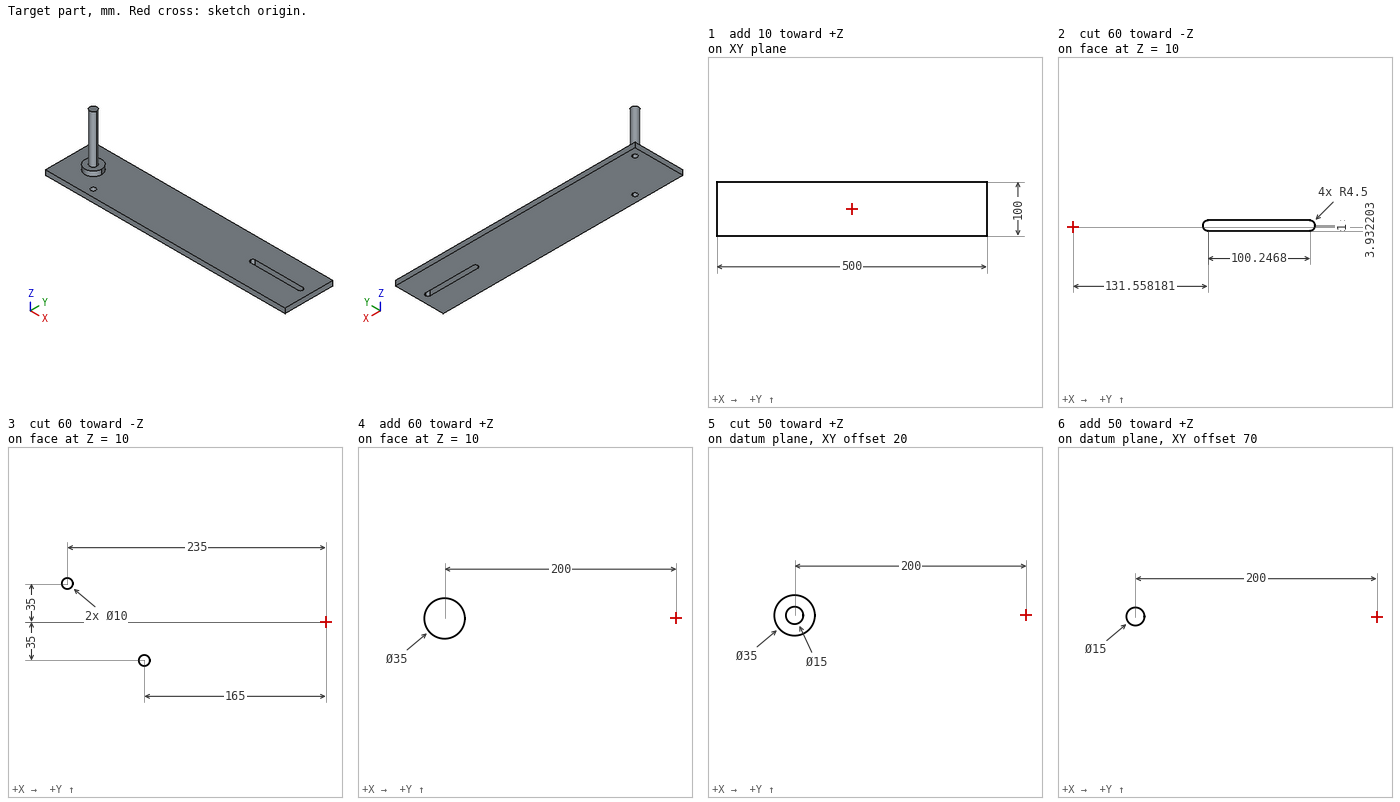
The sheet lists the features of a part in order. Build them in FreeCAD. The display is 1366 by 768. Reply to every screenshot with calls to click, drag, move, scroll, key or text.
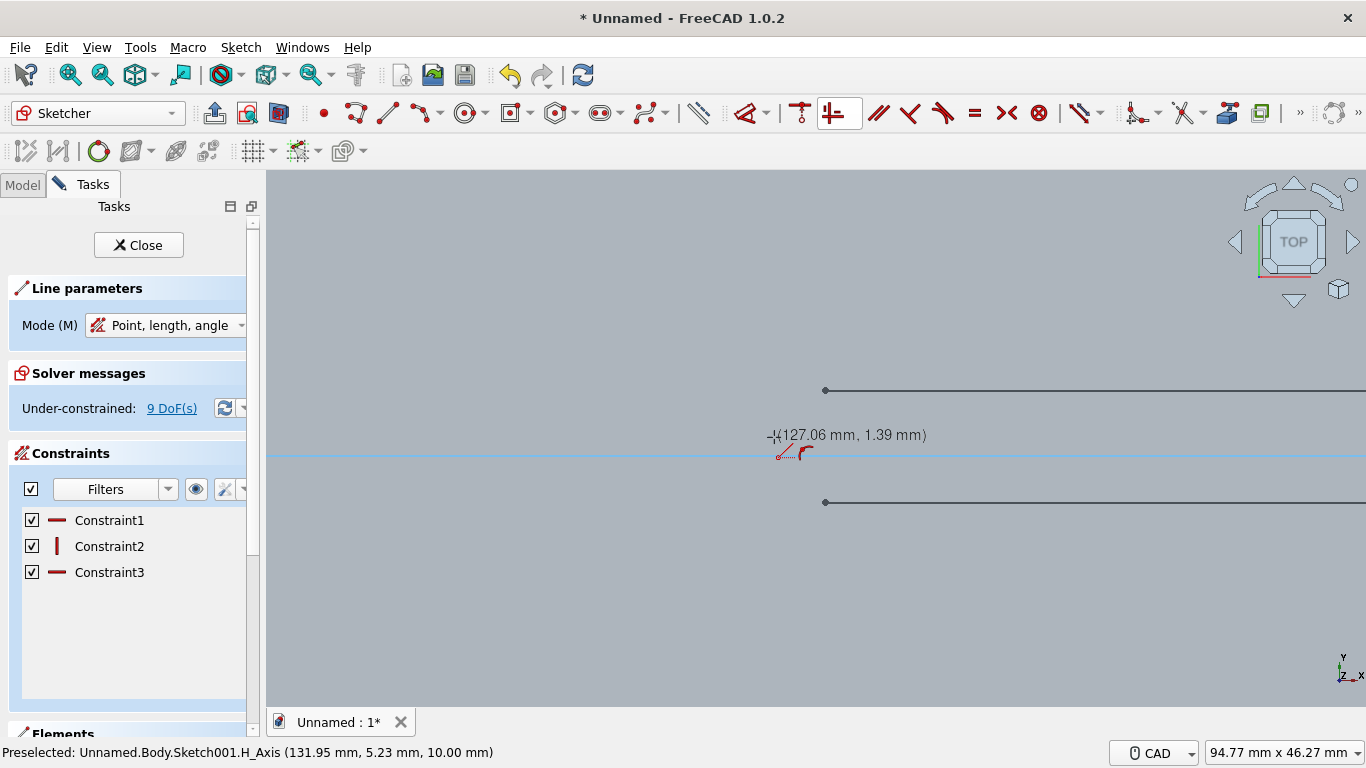
click(773, 437)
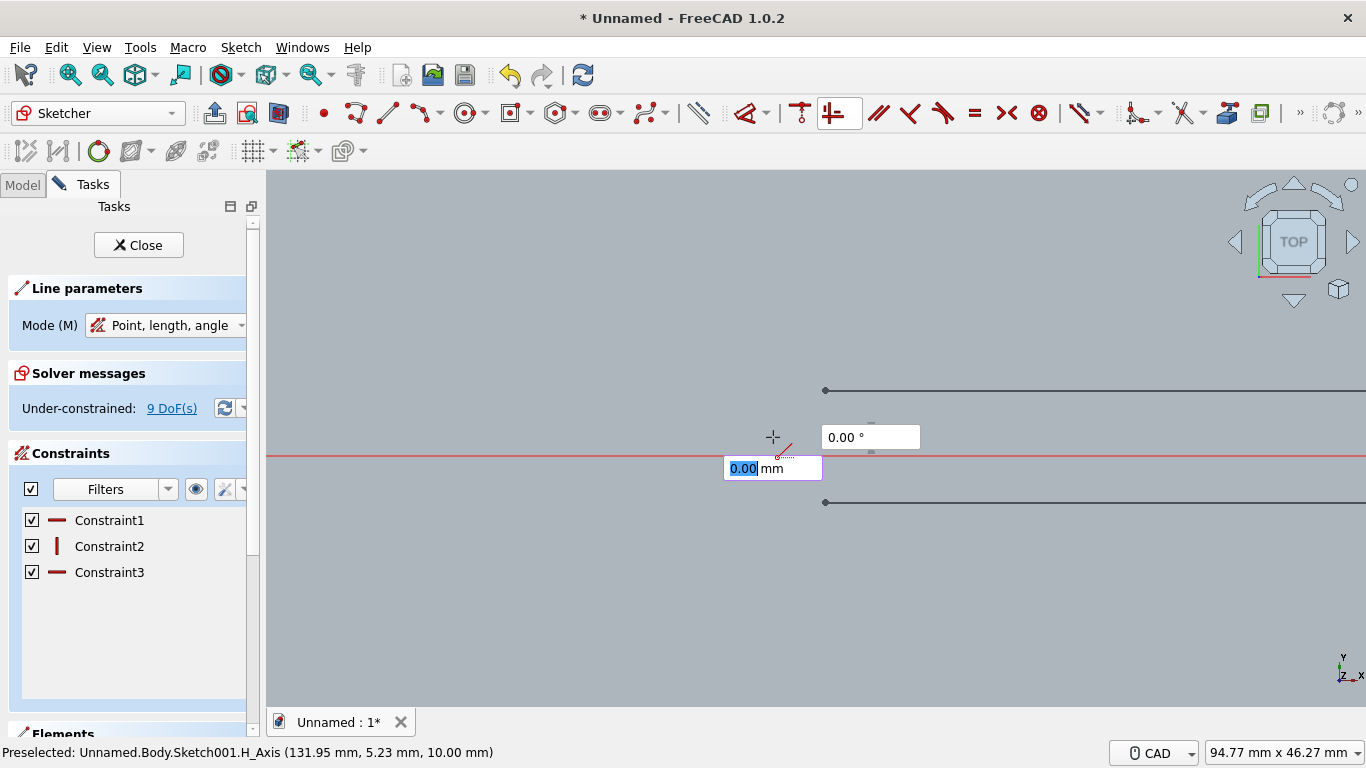
scroll(773, 449, up, 5)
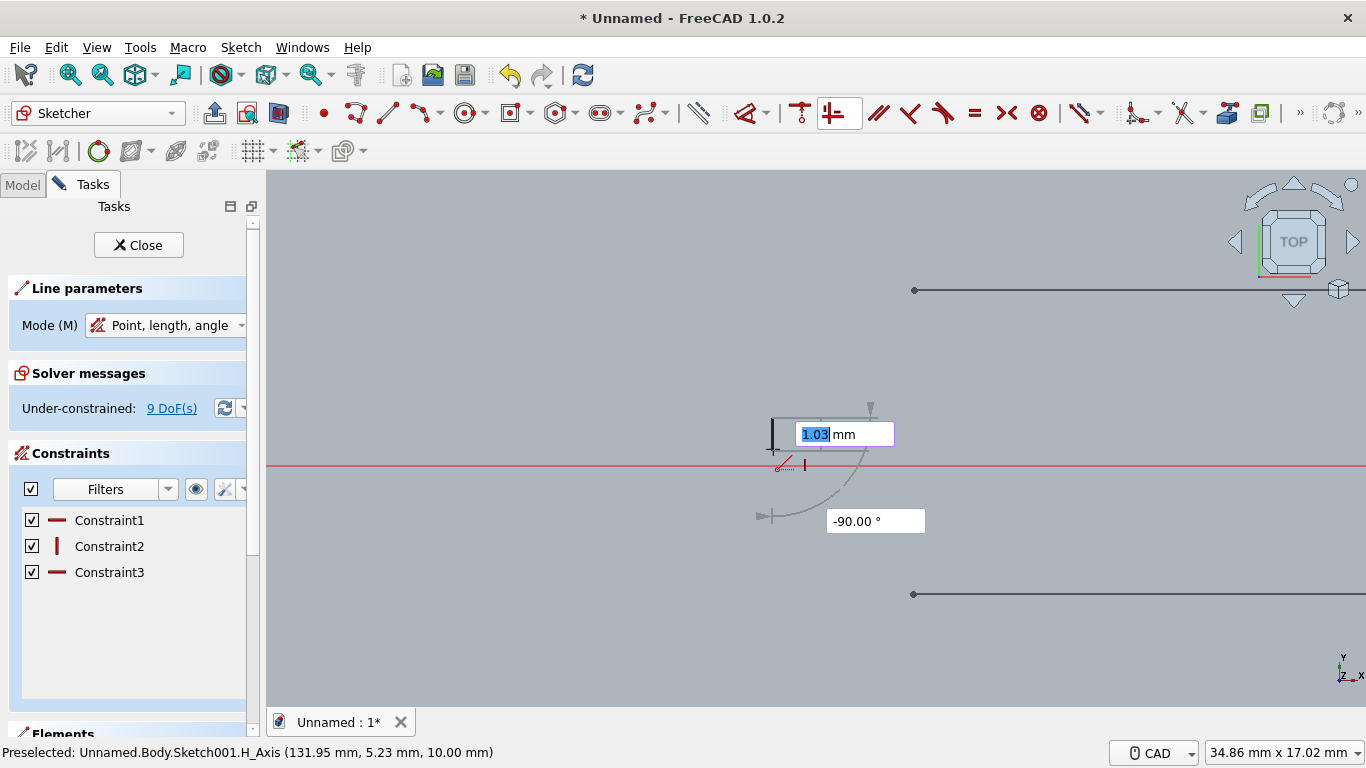
click(772, 448)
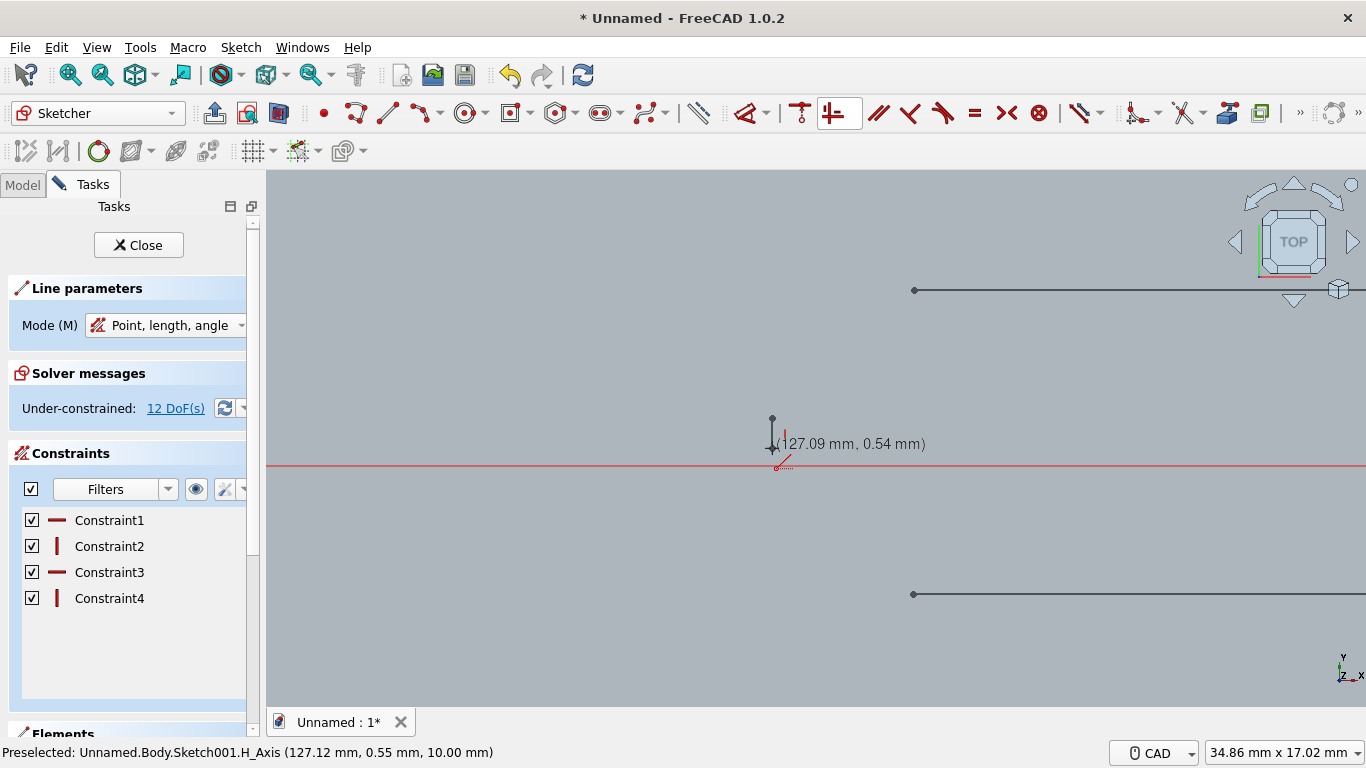
key(g)
key(3)
key(a)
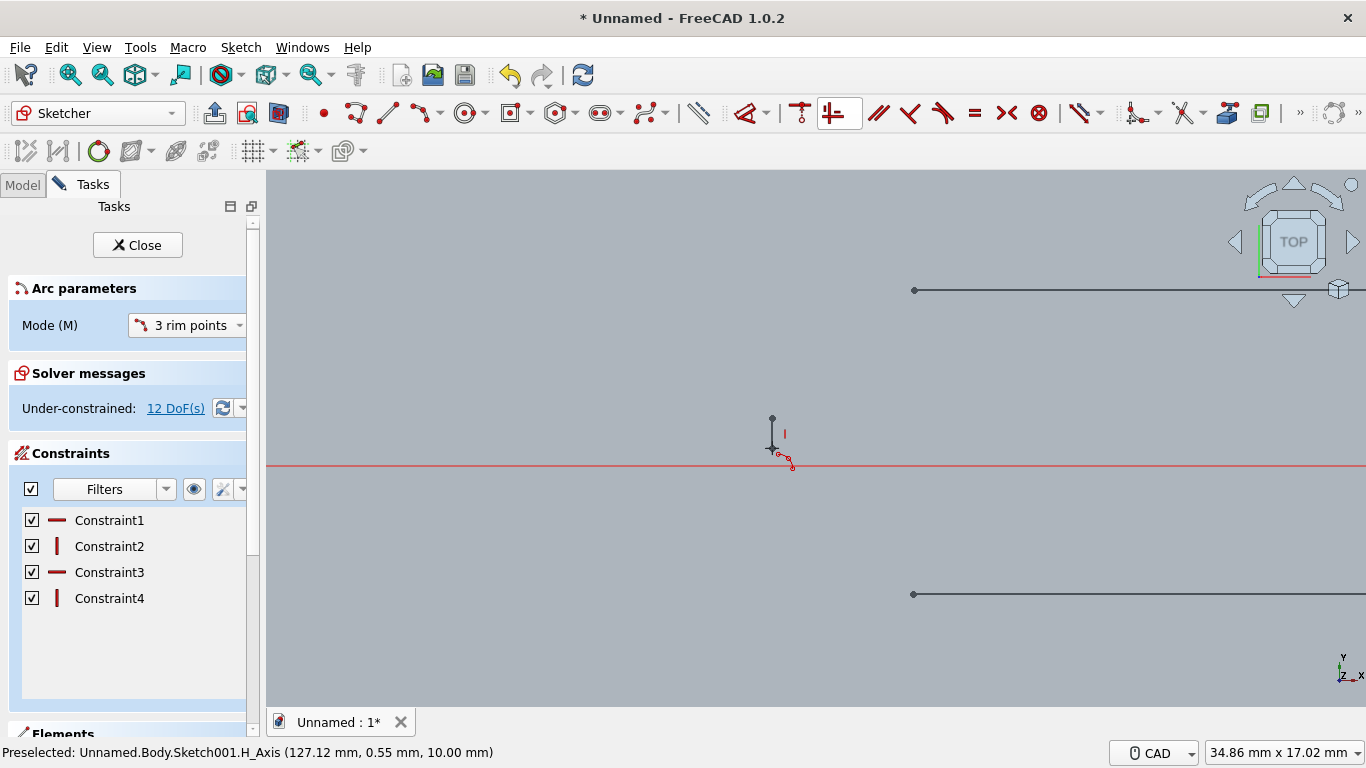
scroll(773, 439, down, 12)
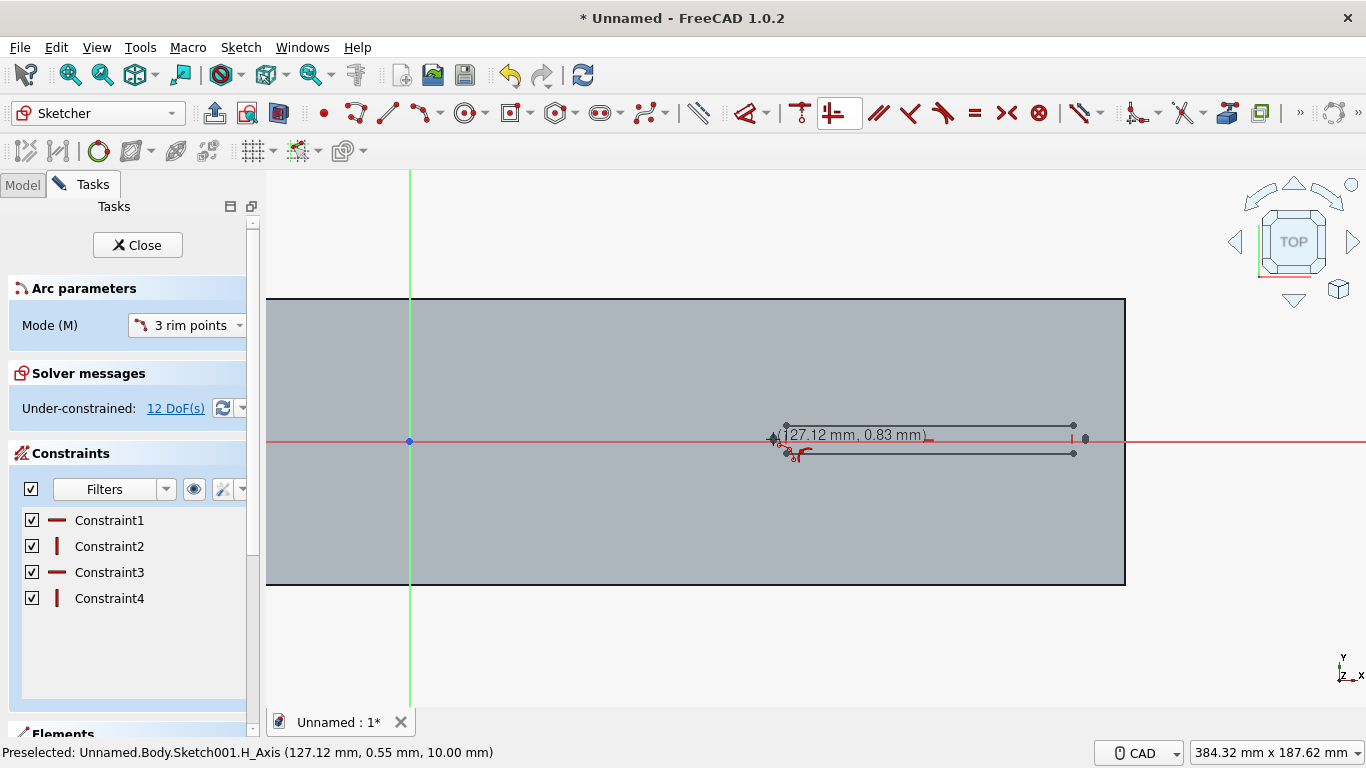
scroll(1073, 453, up, 2)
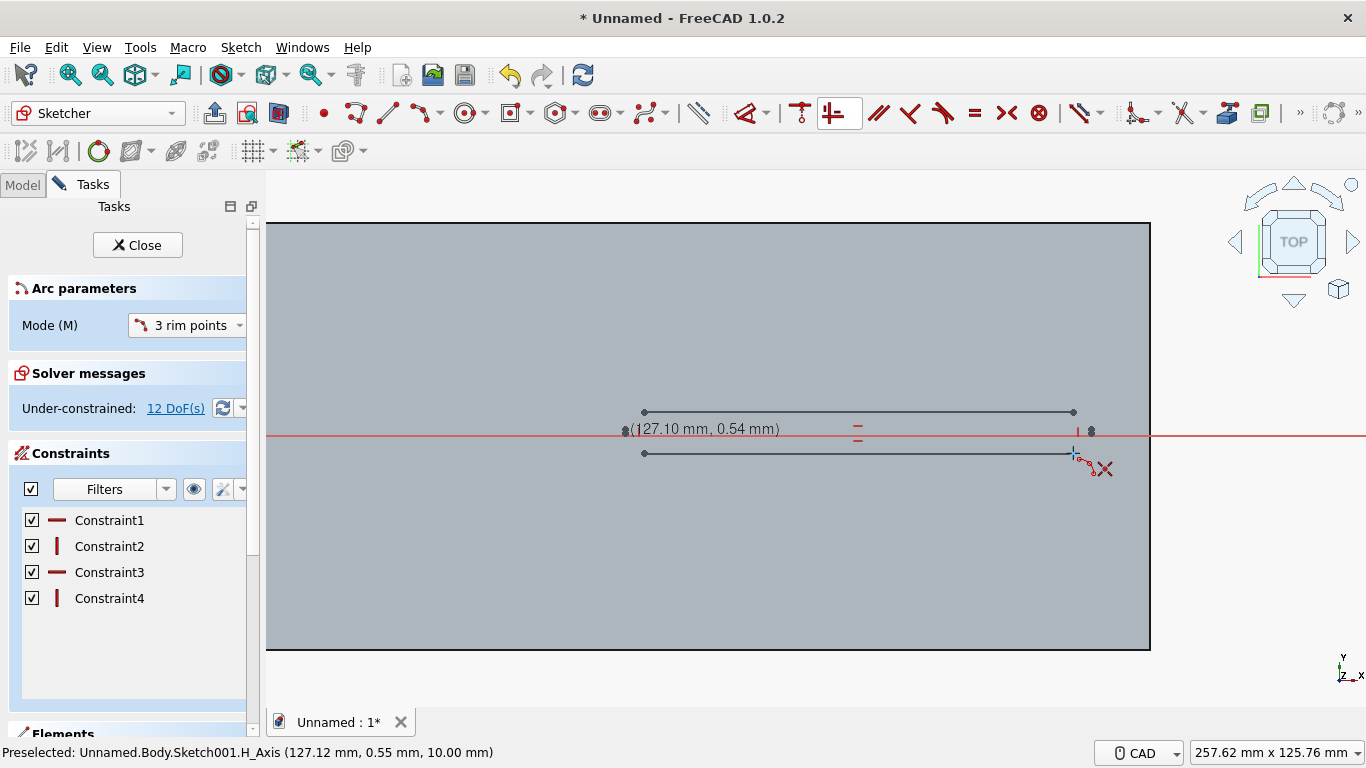
click(1073, 454)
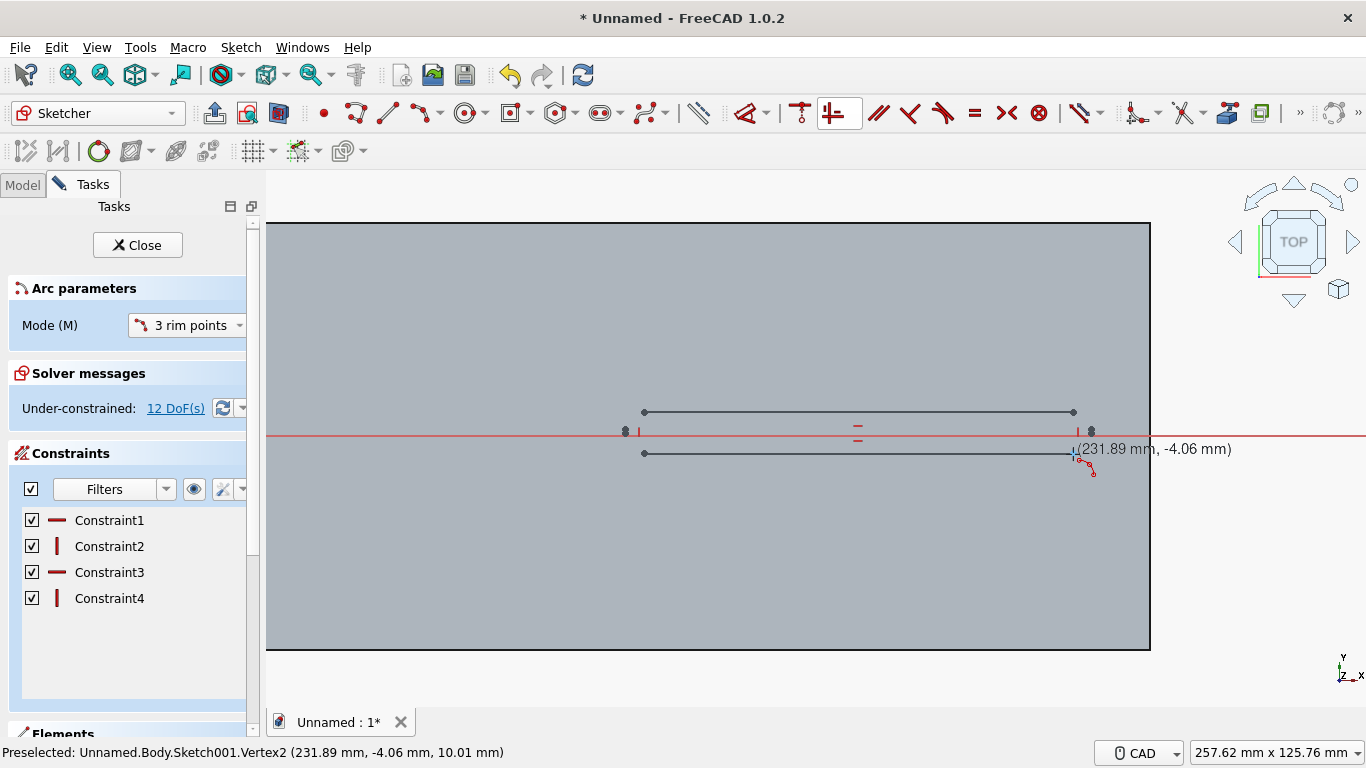
scroll(1092, 434, up, 11)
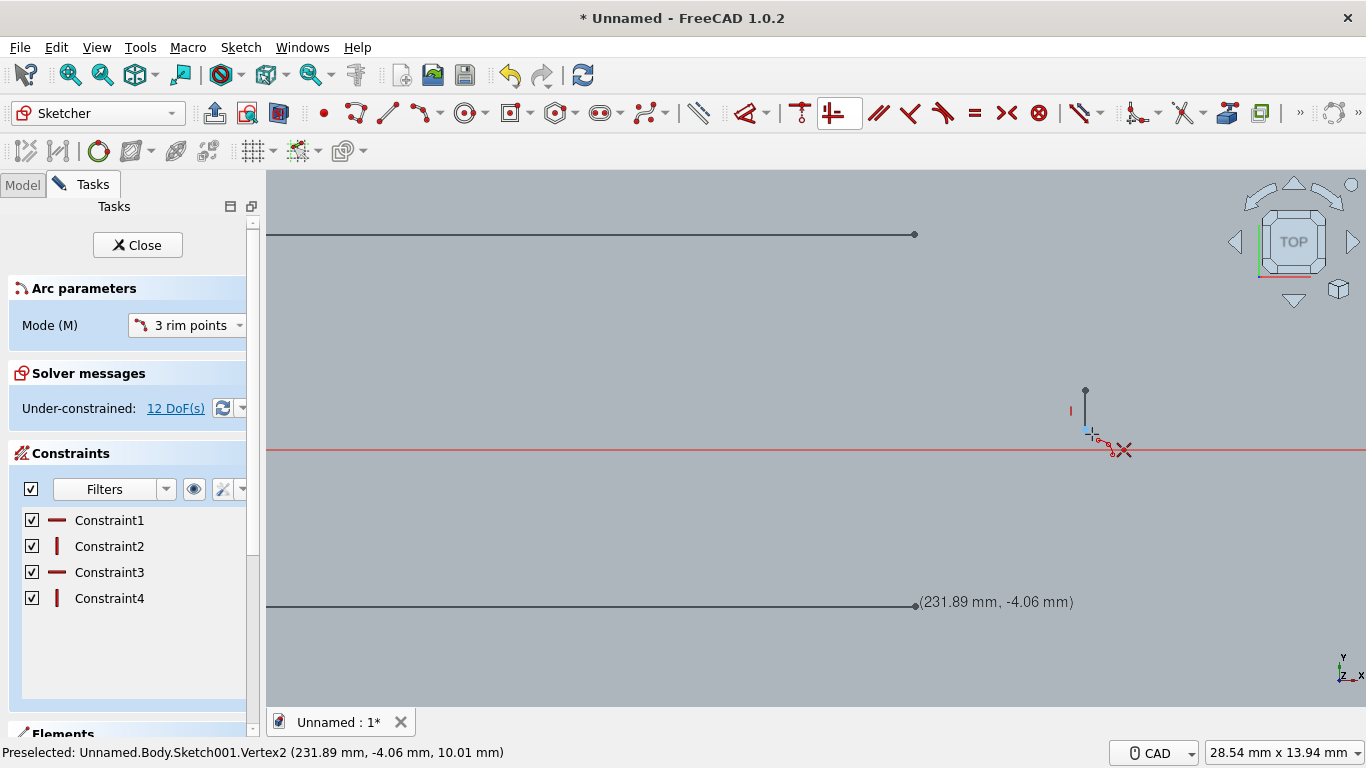
click(1085, 430)